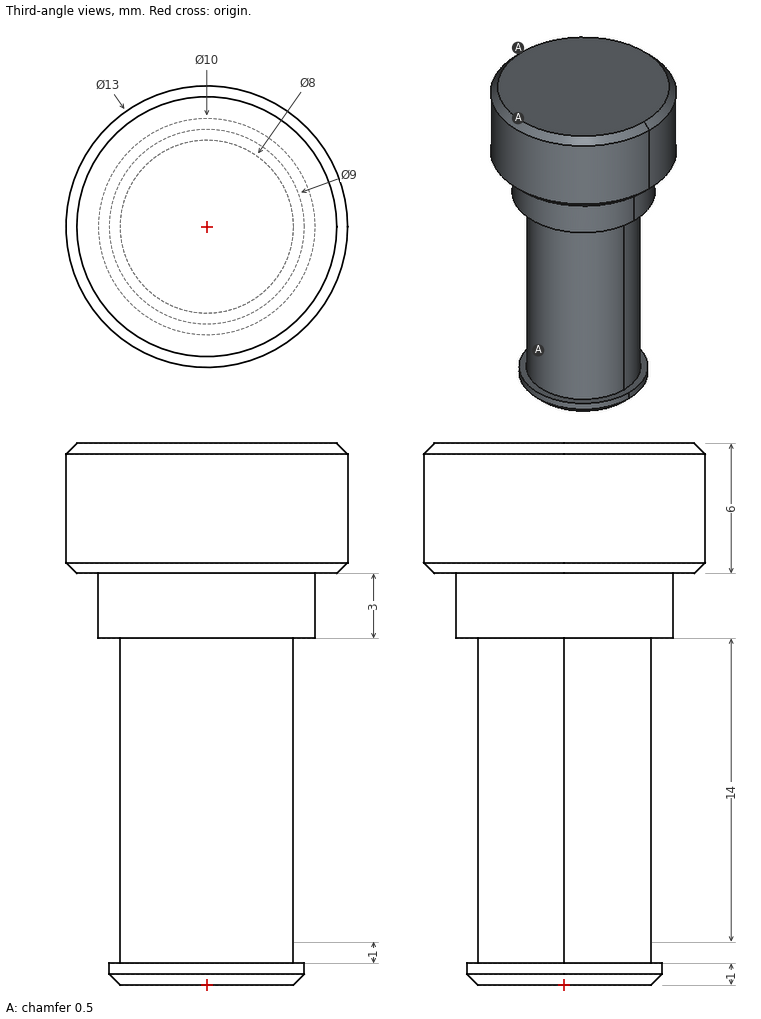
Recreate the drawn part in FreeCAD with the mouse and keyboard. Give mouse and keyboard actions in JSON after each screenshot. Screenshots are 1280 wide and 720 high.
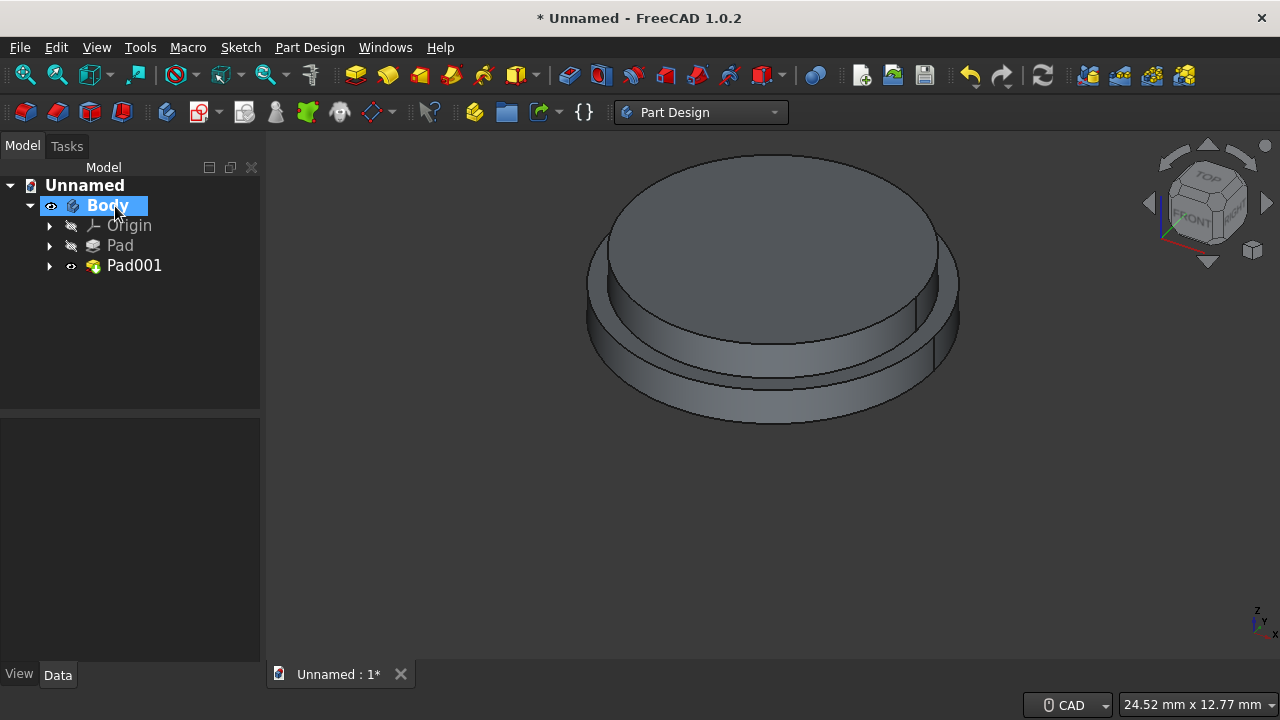
{"action": "left_click", "coordinate": [26, 76]}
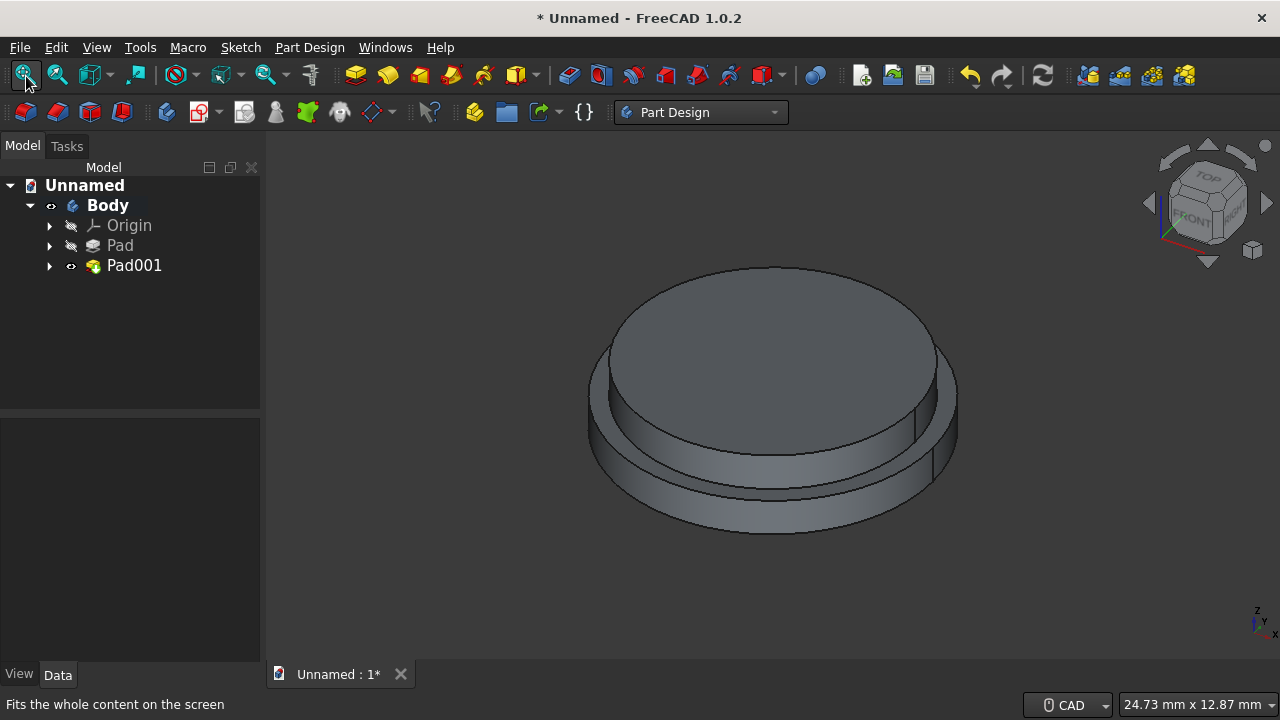
{"action": "left_click", "coordinate": [773, 360]}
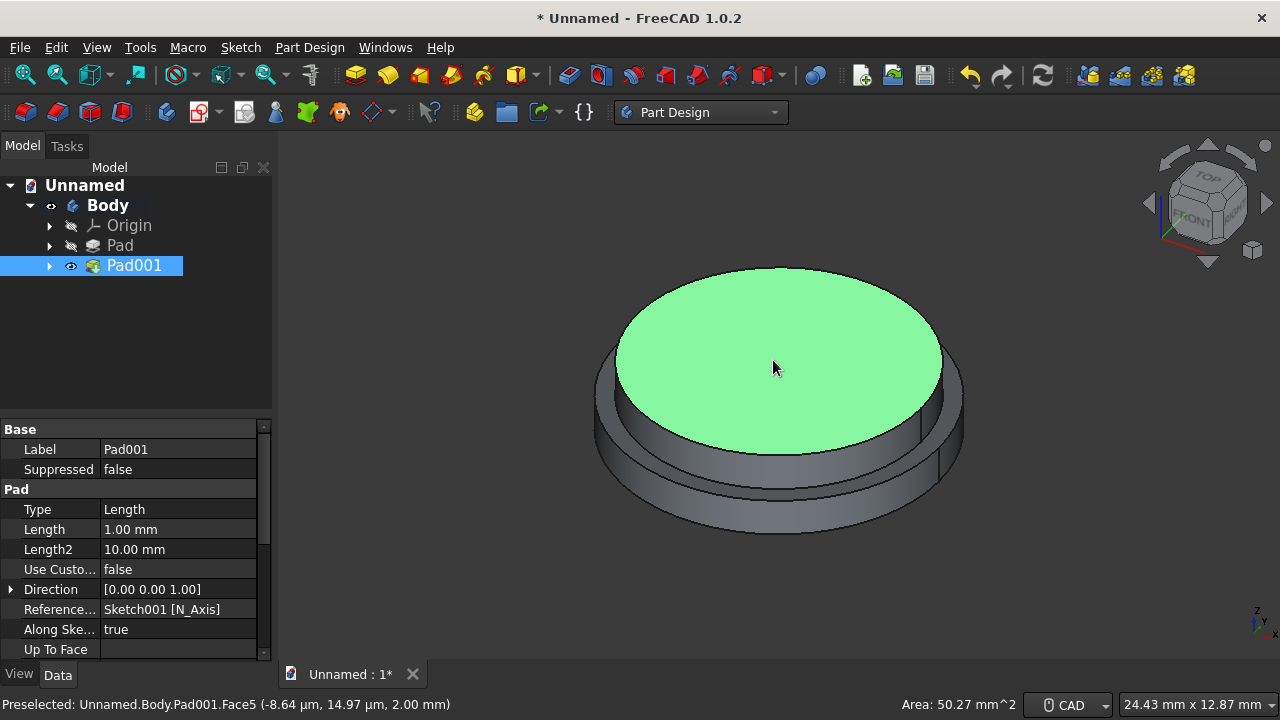
{"action": "left_click", "coordinate": [200, 112]}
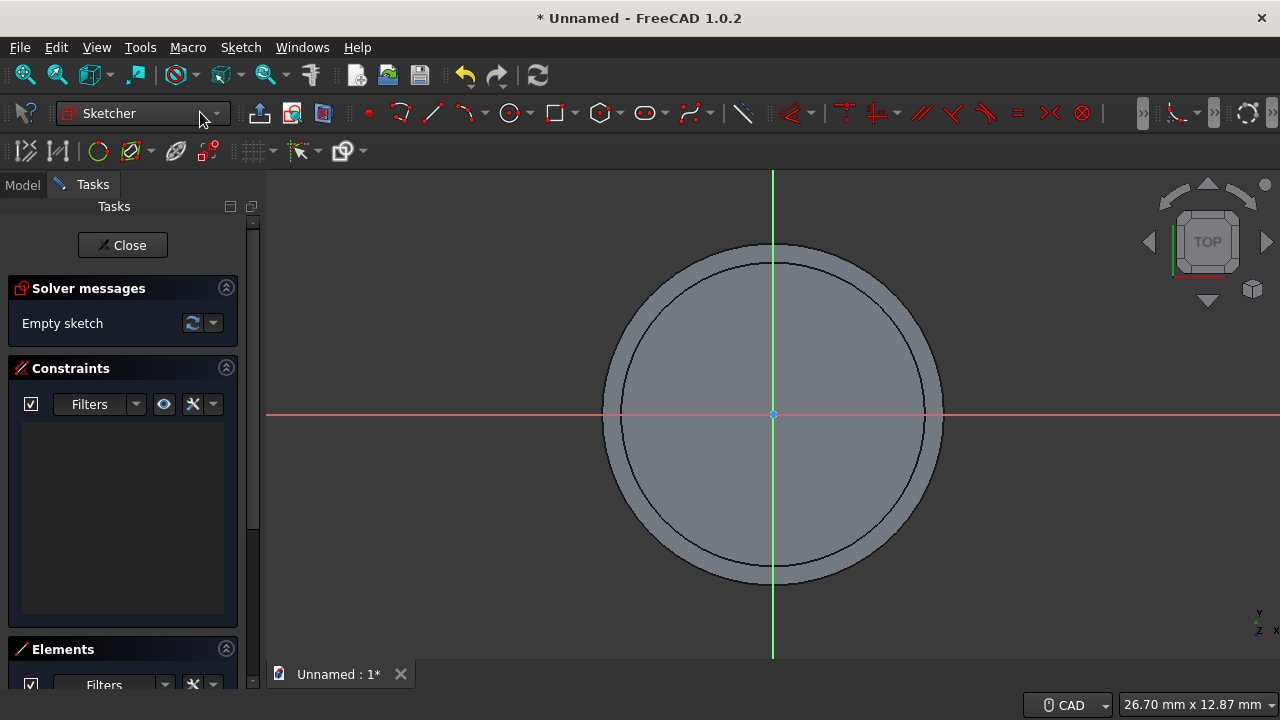
{"action": "left_click", "coordinate": [510, 114]}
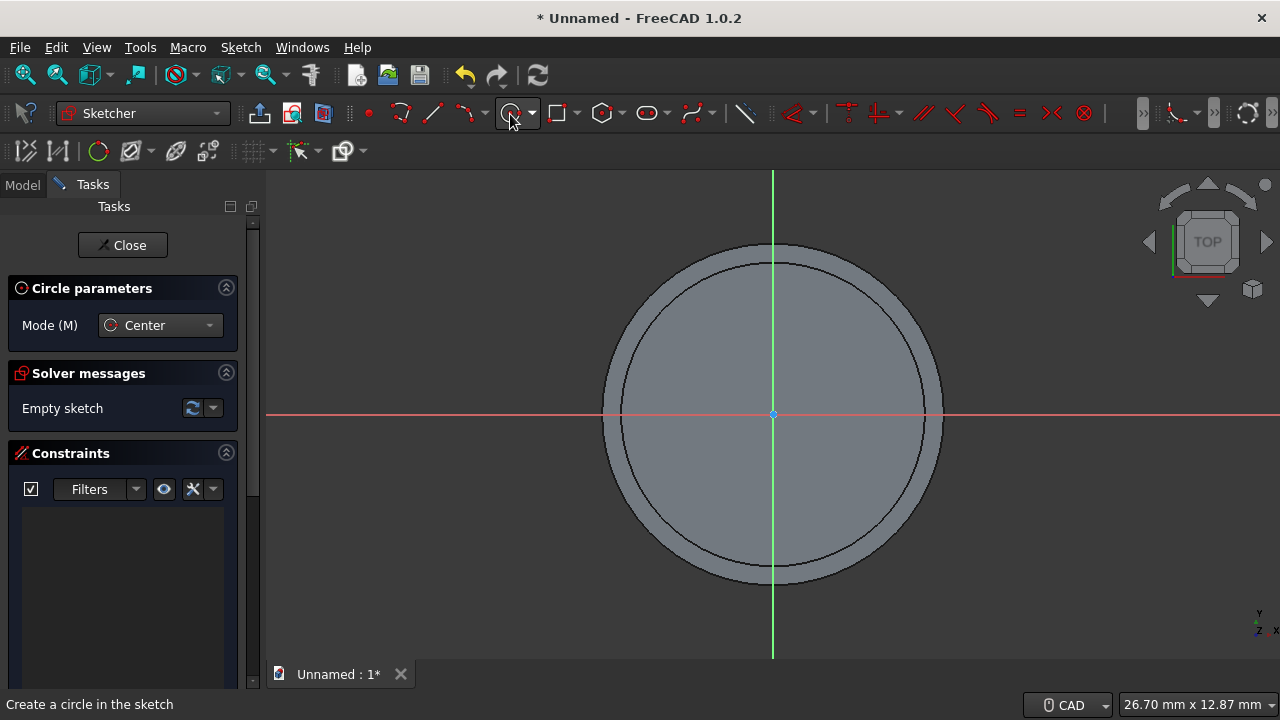
{"action": "left_click", "coordinate": [773, 414]}
{"action": "mouse_move", "coordinate": [880, 307]}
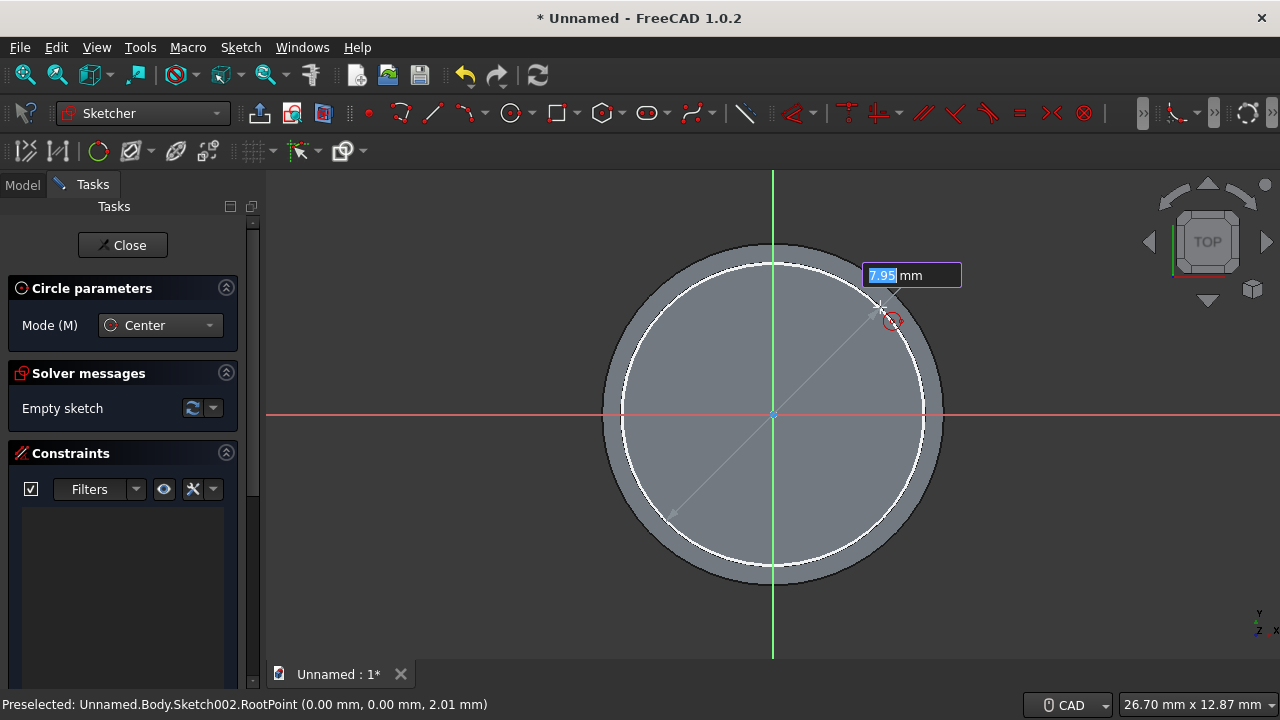
{"action": "type", "text": "8"}
{"action": "key", "text": "Return"}
{"action": "key", "text": "Escape"}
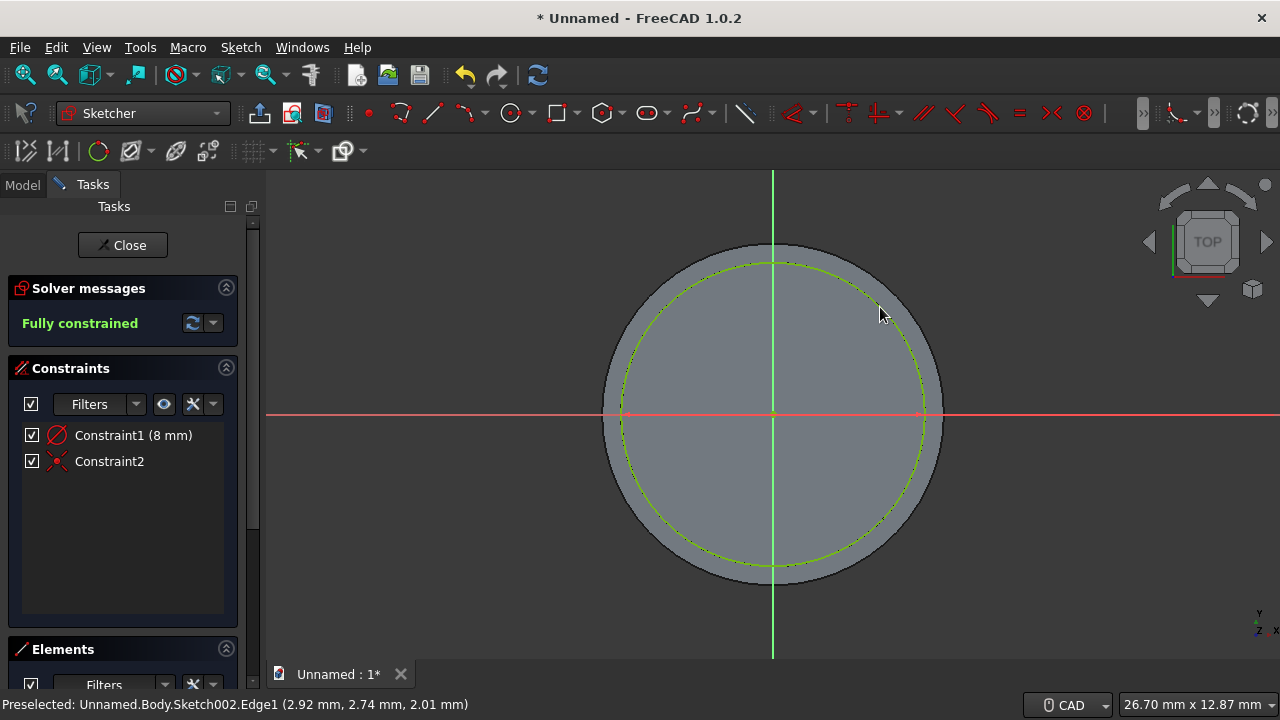
{"action": "left_click", "coordinate": [123, 245]}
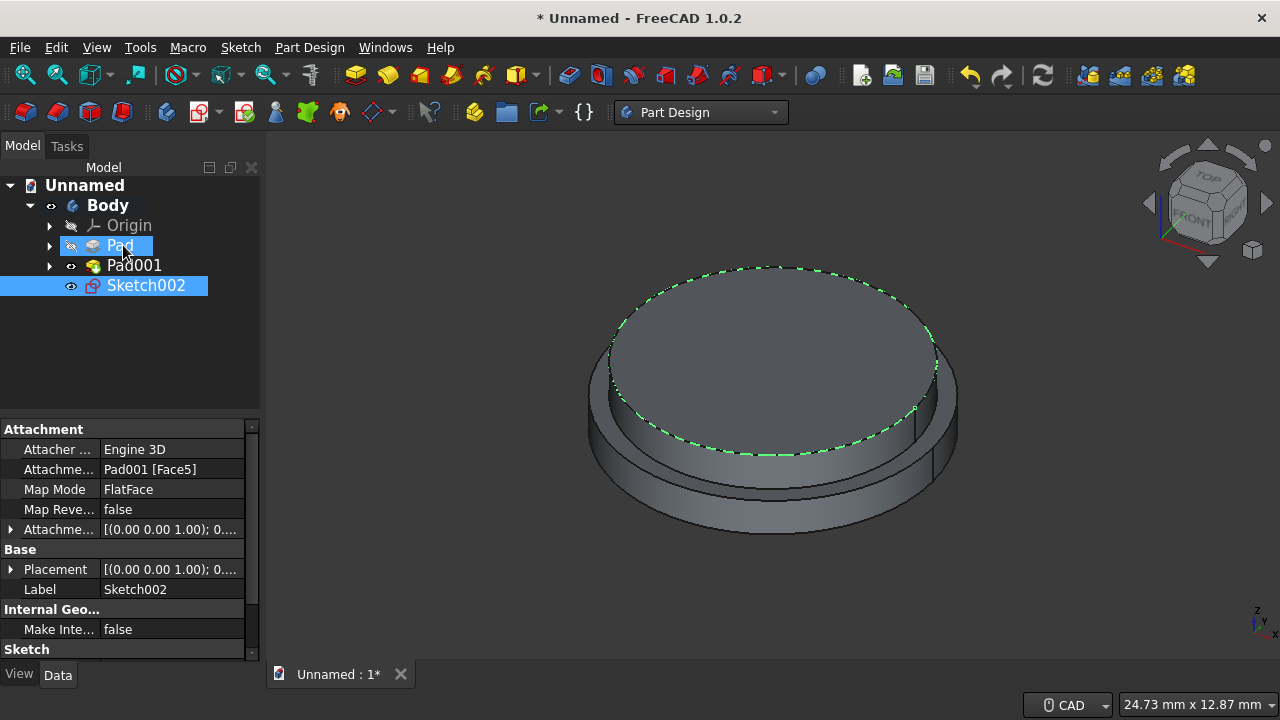
{"action": "left_click", "coordinate": [356, 76]}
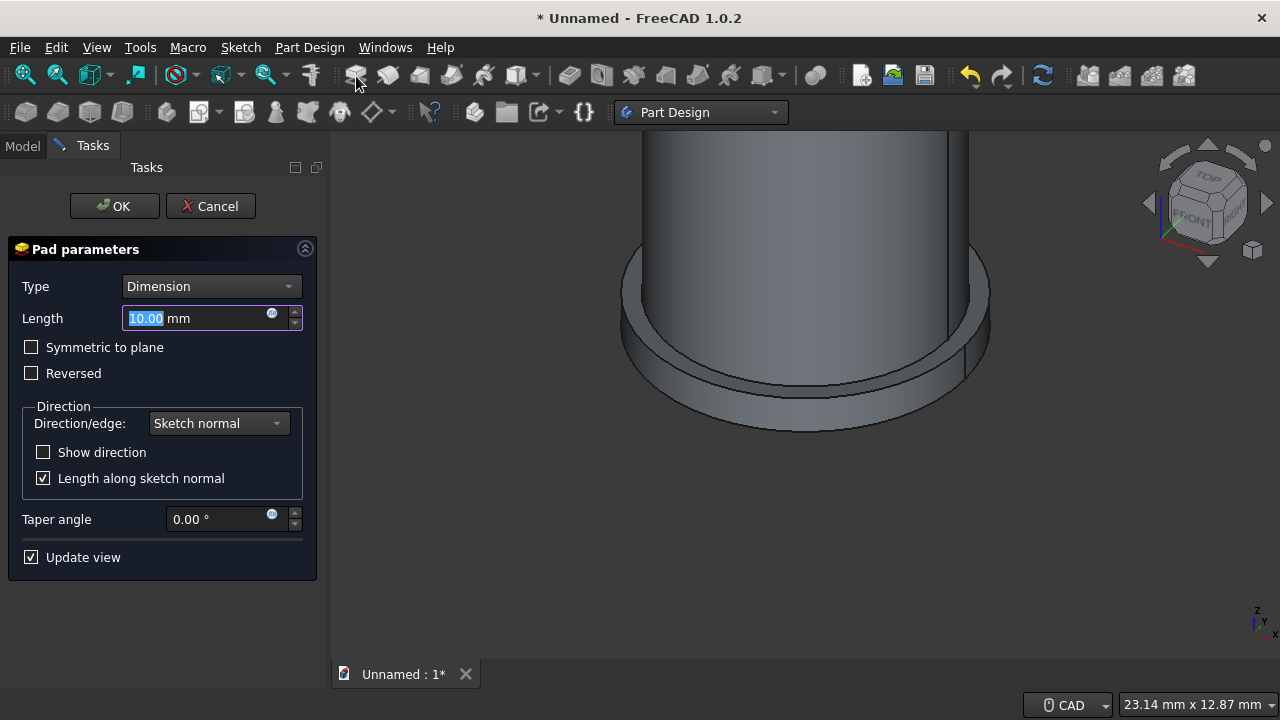
{"action": "type", "text": "14"}
{"action": "key", "text": "Tab"}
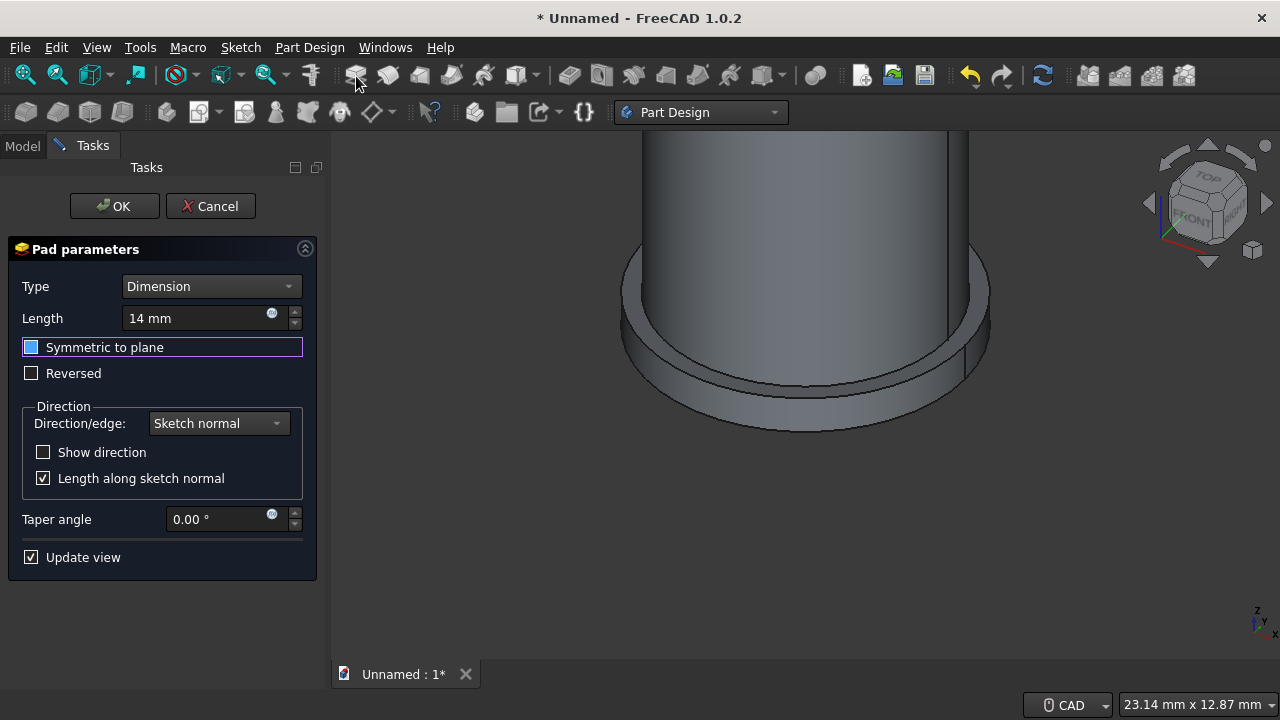
{"action": "left_click", "coordinate": [115, 206]}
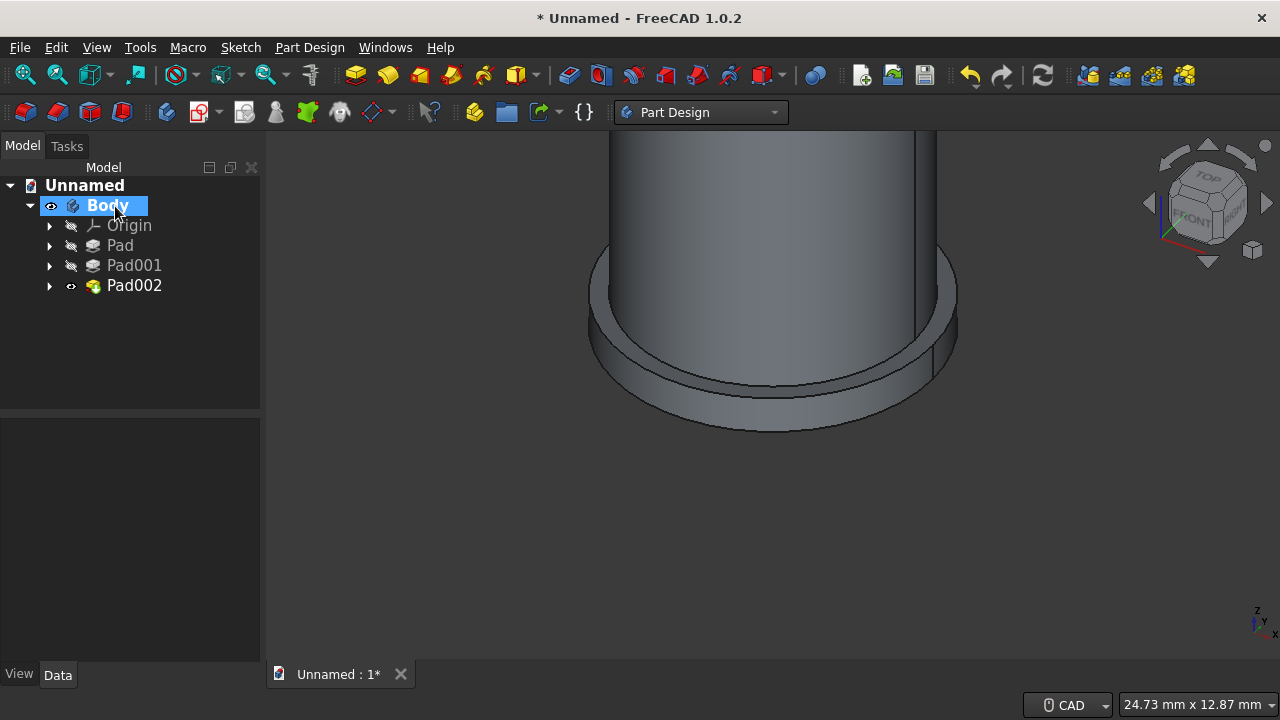
{"action": "left_click", "coordinate": [26, 76]}